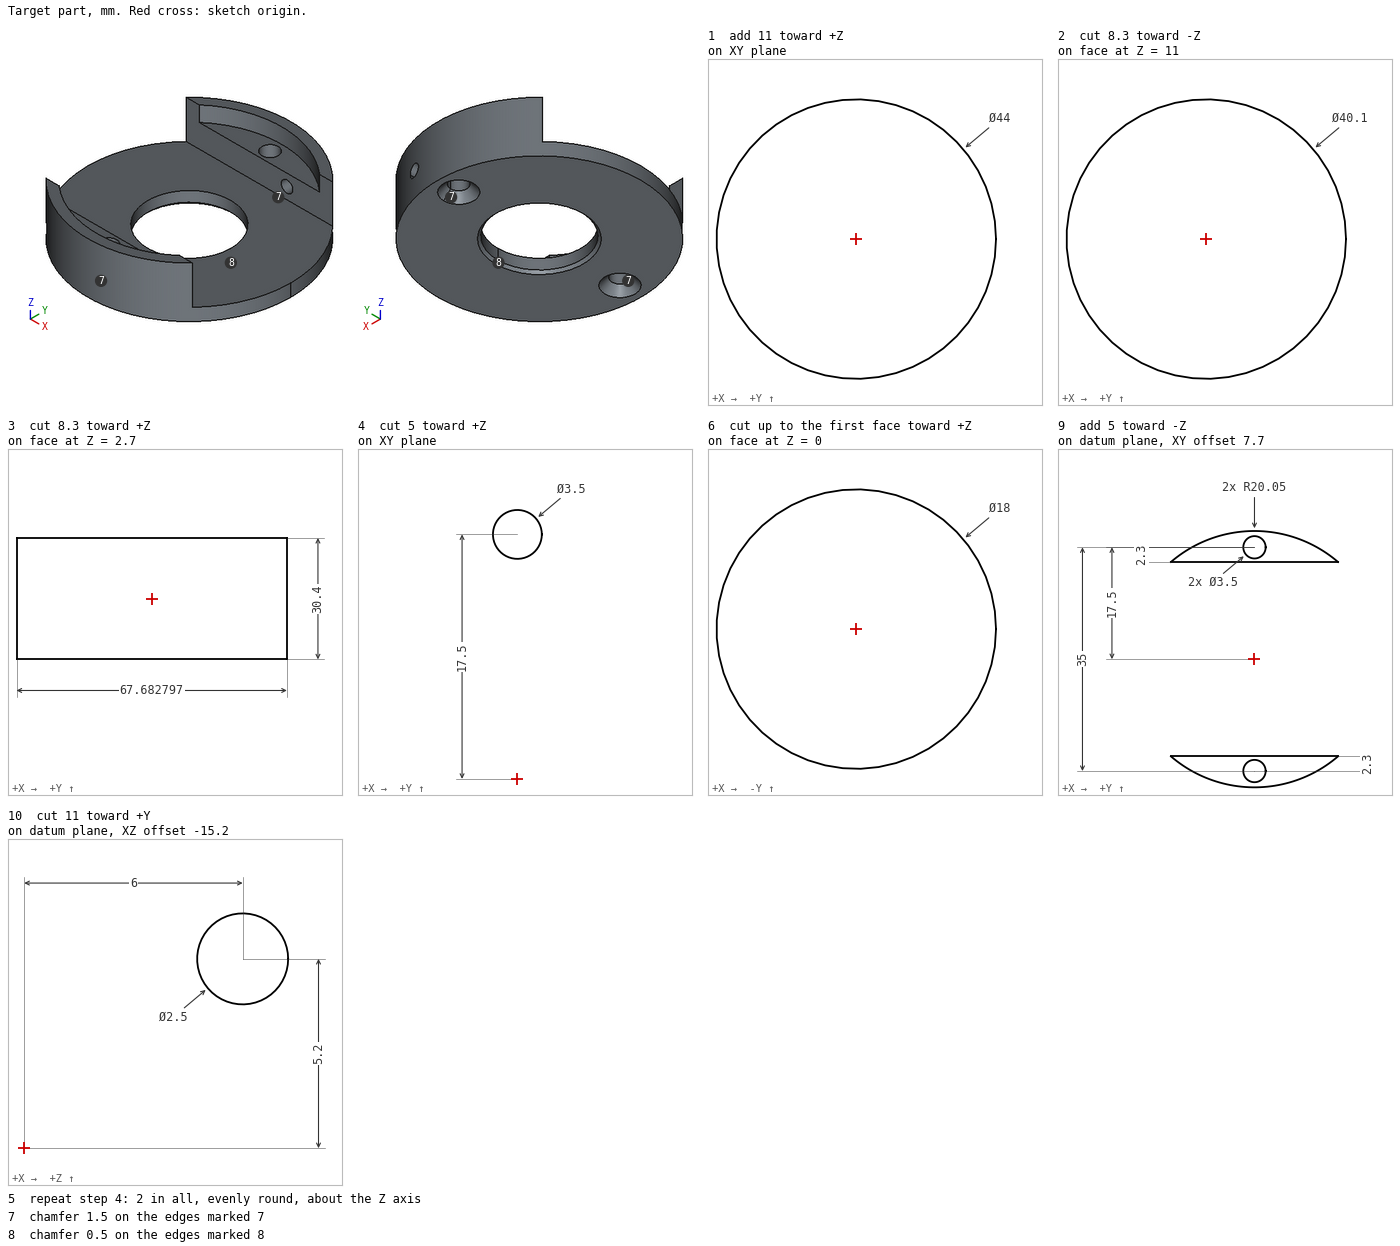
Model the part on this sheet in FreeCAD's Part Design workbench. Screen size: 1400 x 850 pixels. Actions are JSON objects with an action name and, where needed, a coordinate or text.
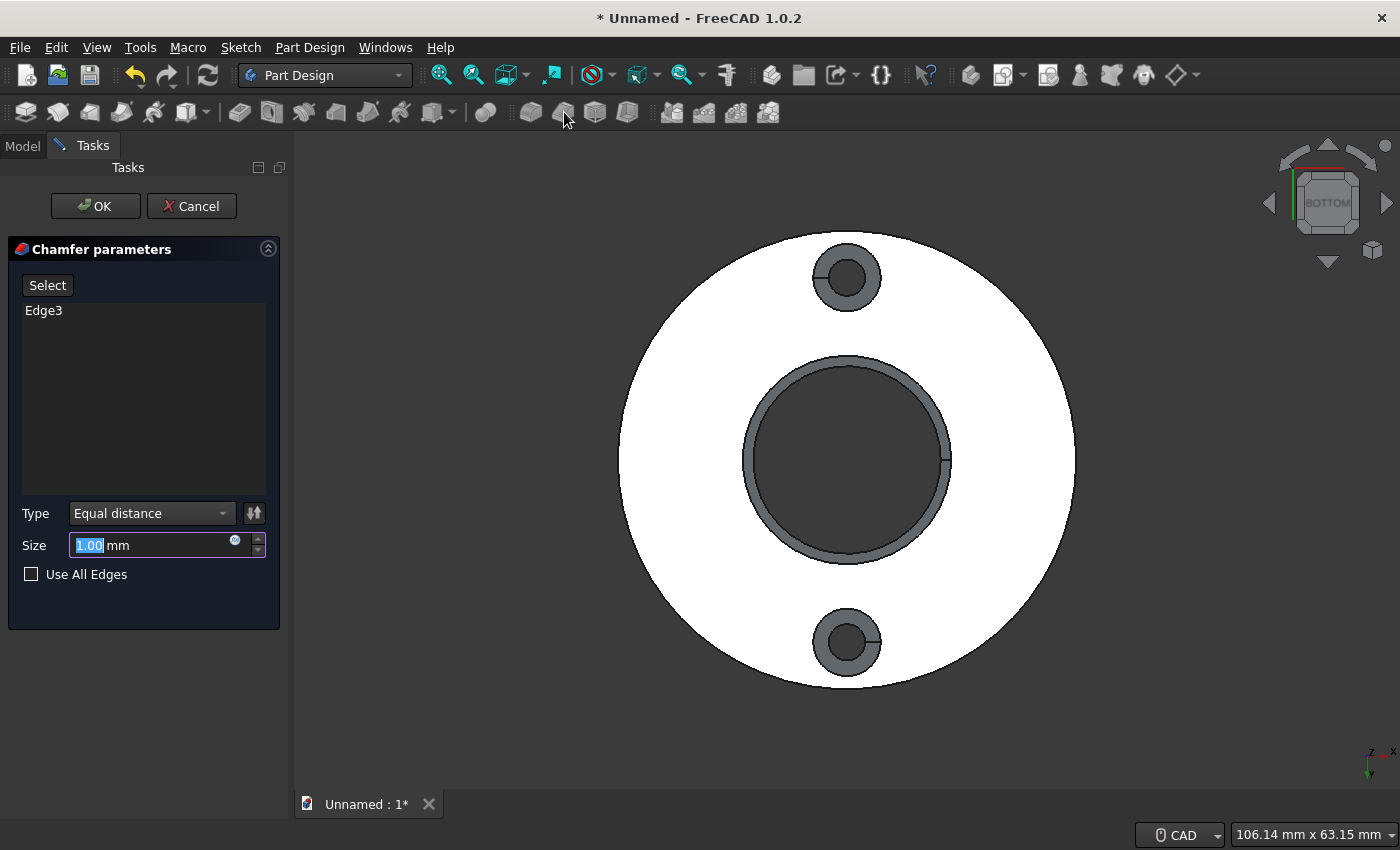
{"action": "type", "text": "0.5"}
{"action": "key", "text": "Tab"}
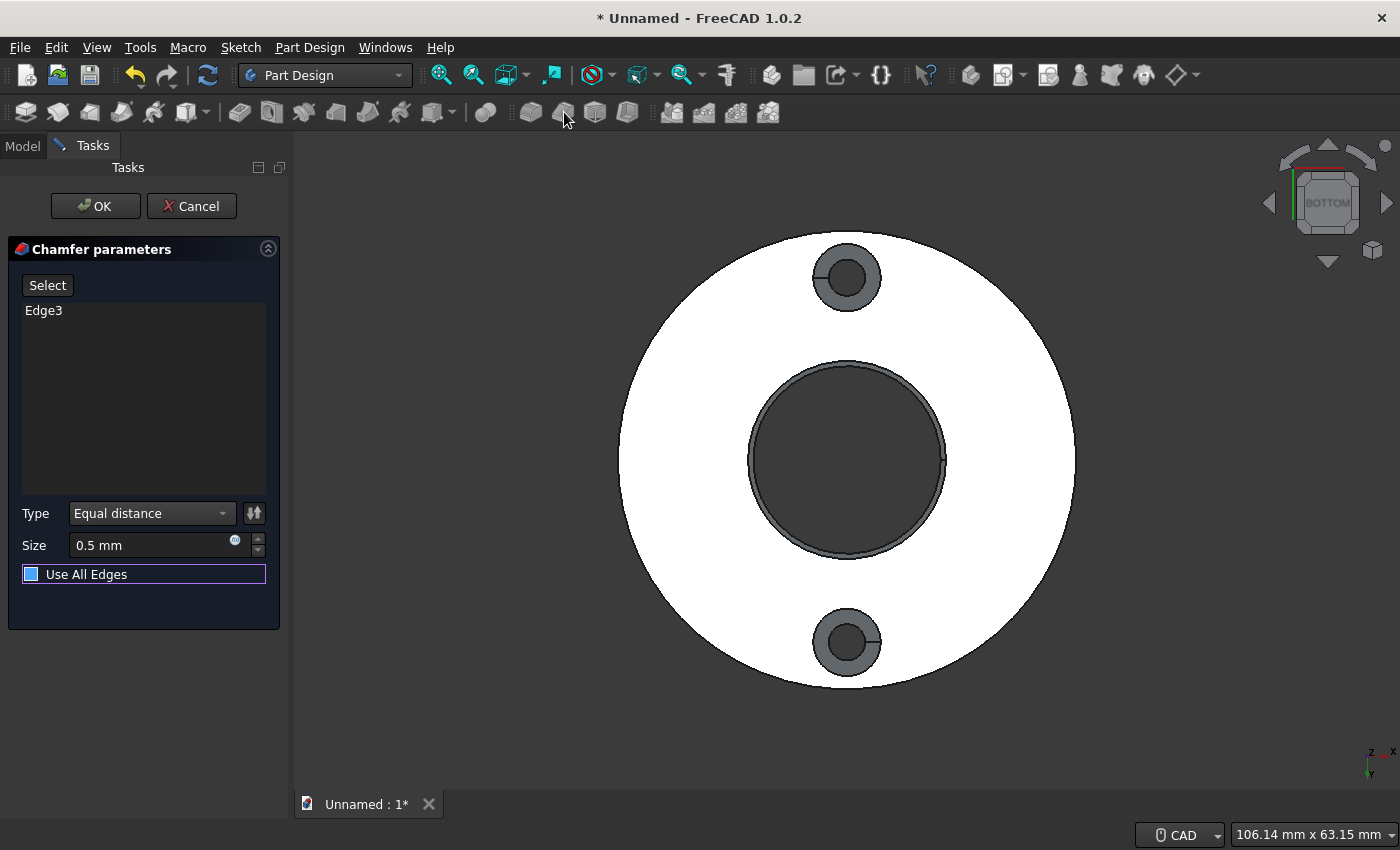
{"action": "left_click", "coordinate": [96, 206]}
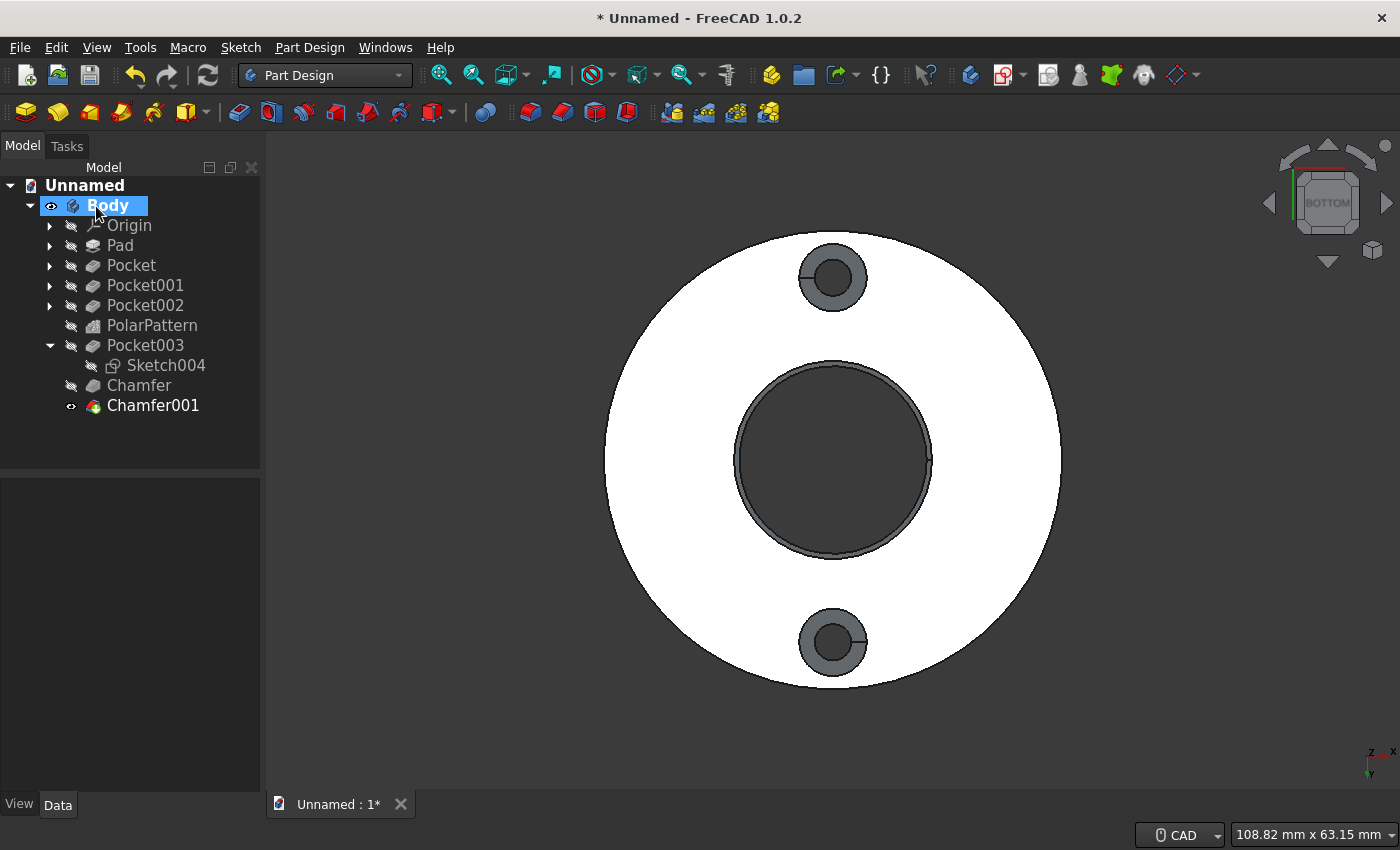
{"action": "left_click", "coordinate": [50, 226]}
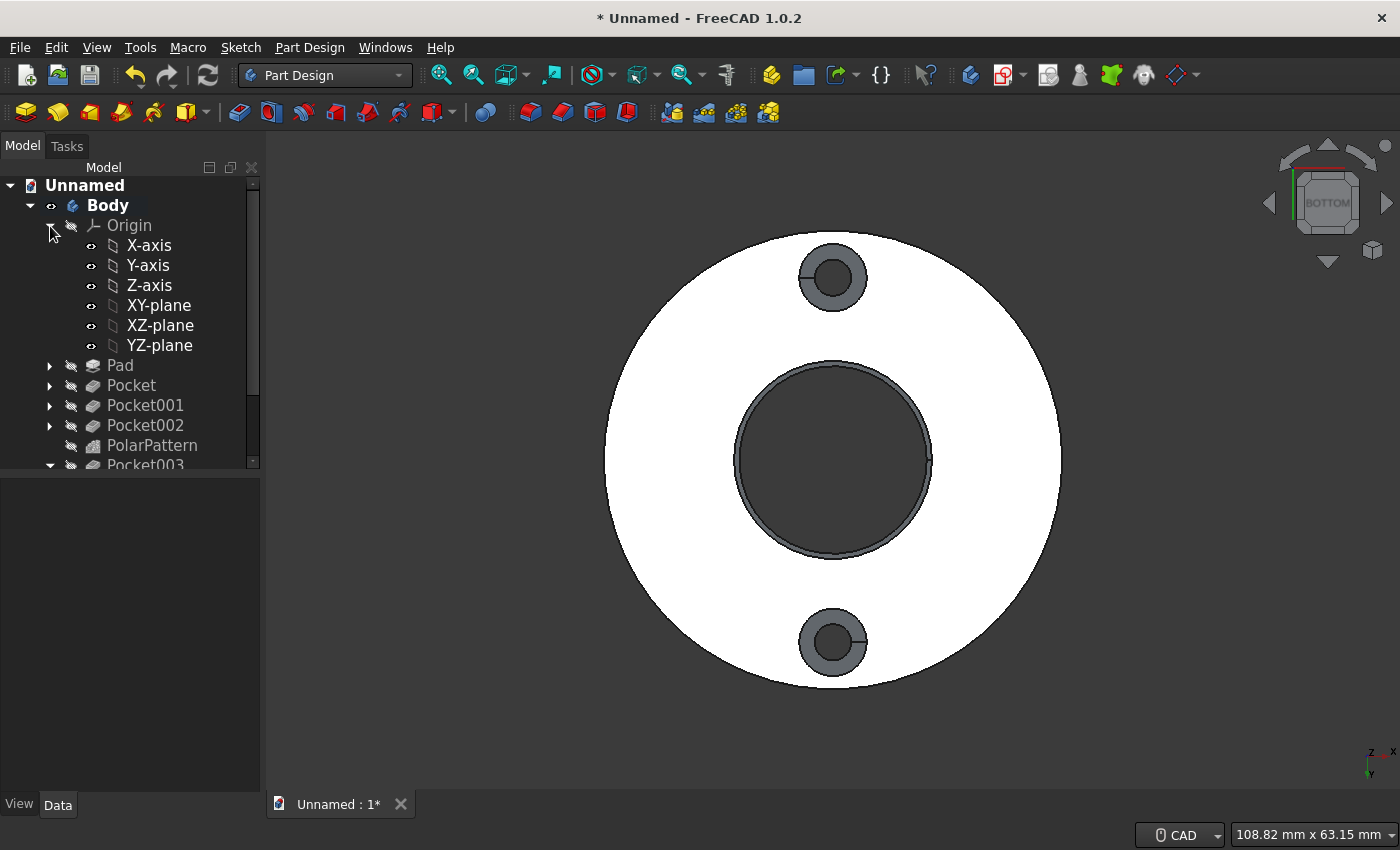
{"action": "left_click", "coordinate": [136, 306]}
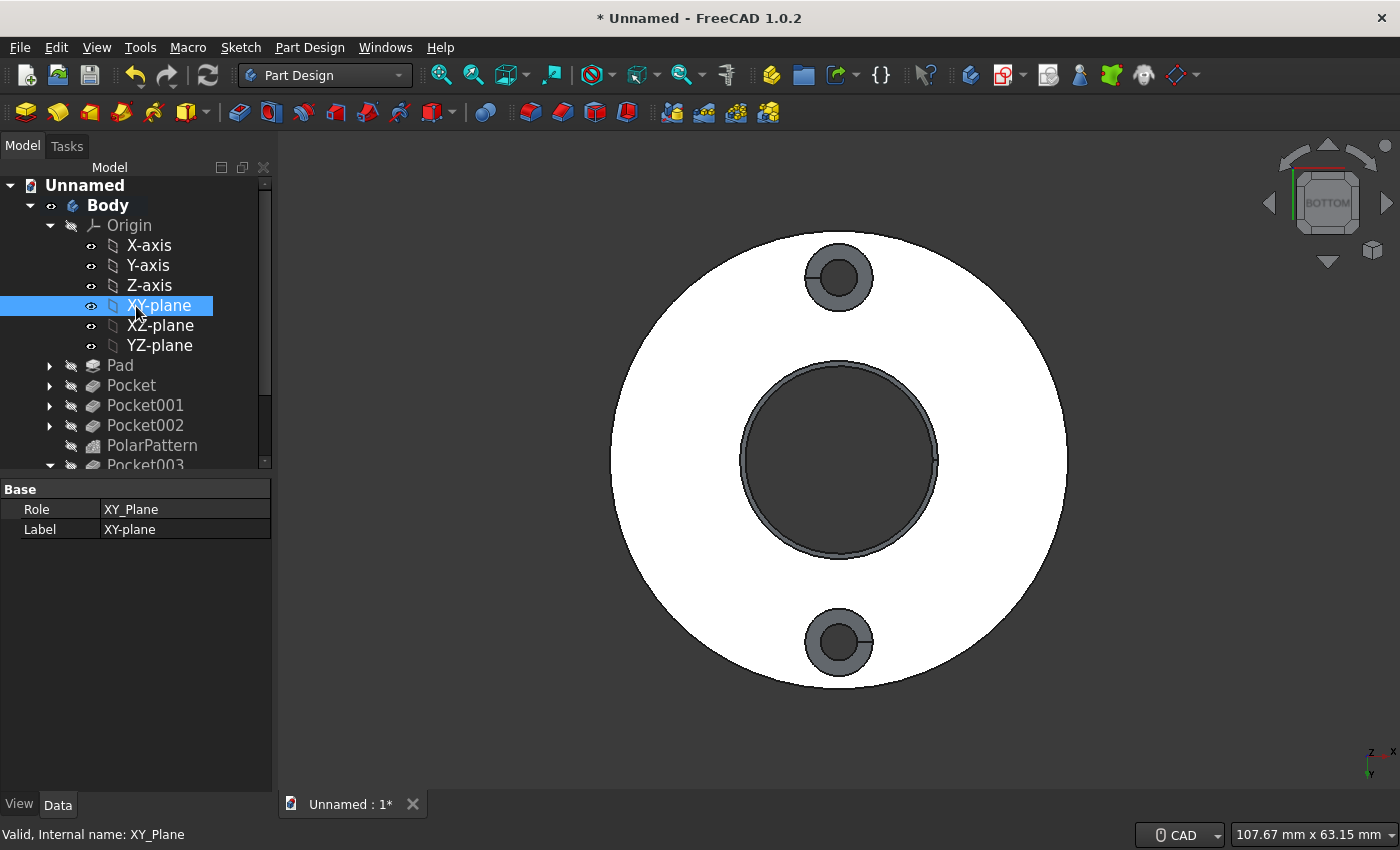
{"action": "left_click", "coordinate": [1176, 76]}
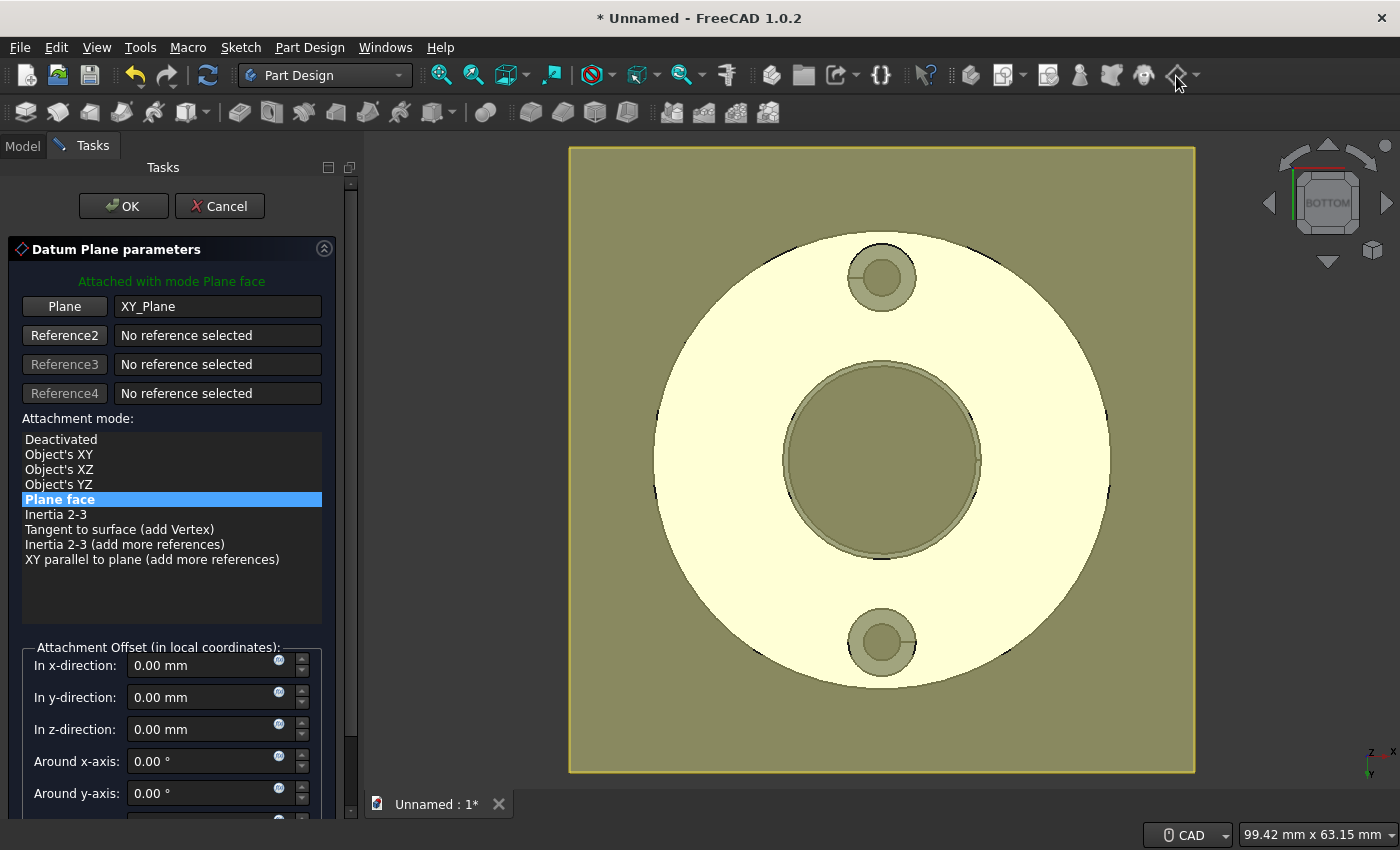
{"action": "triple_click", "coordinate": [210, 729]}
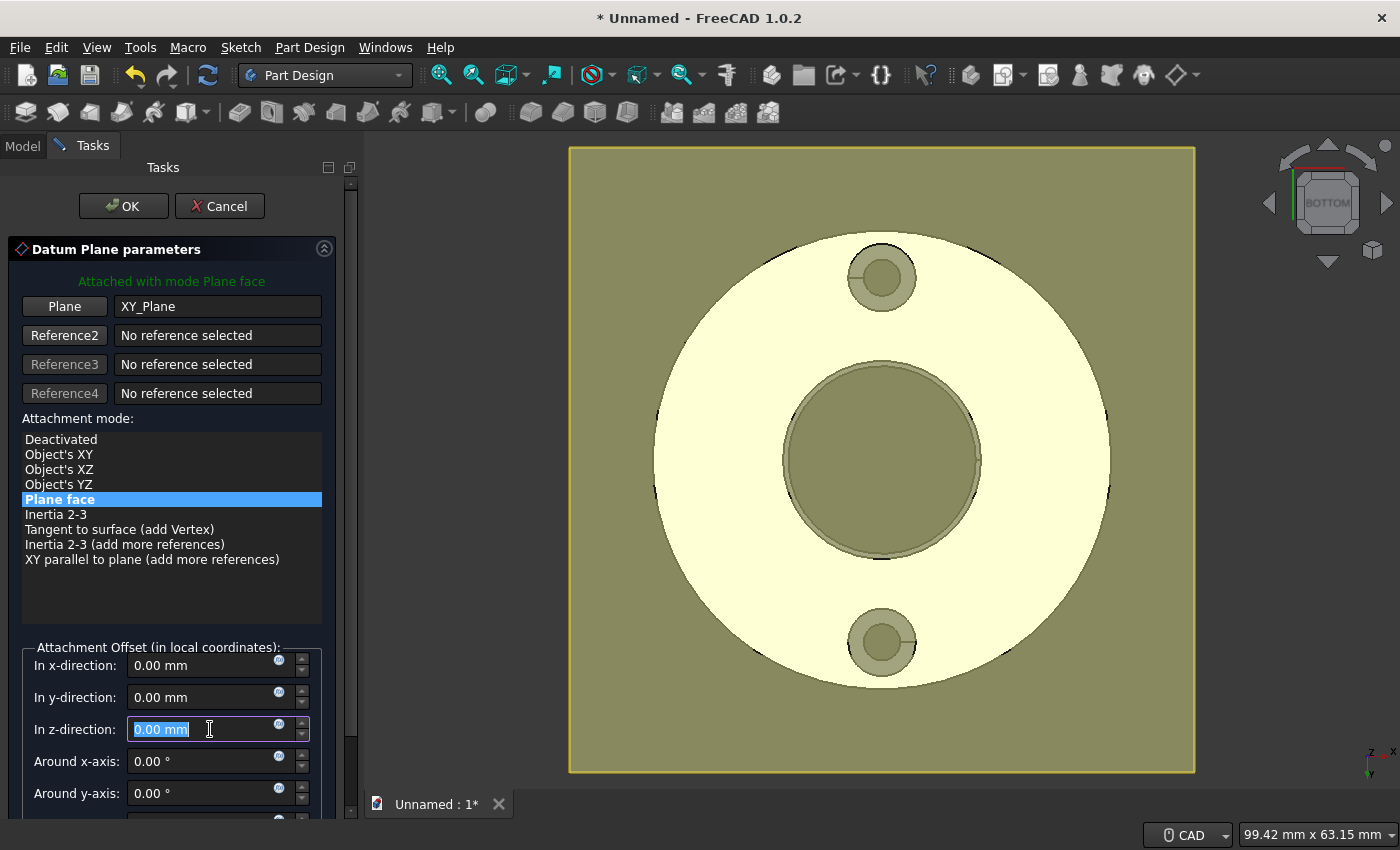
{"action": "type", "text": "7.7"}
{"action": "key", "text": "Tab"}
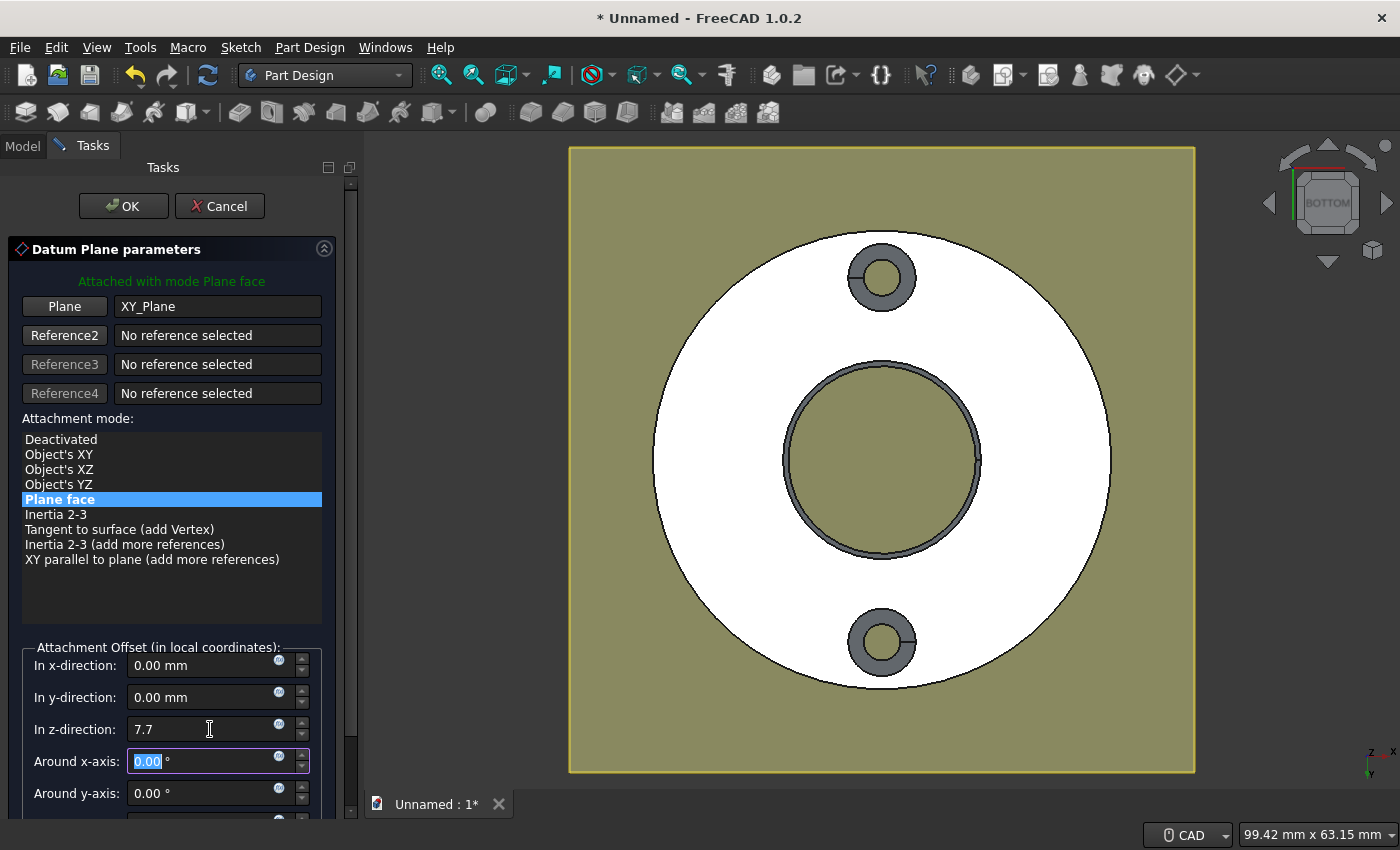
{"action": "left_click", "coordinate": [124, 206]}